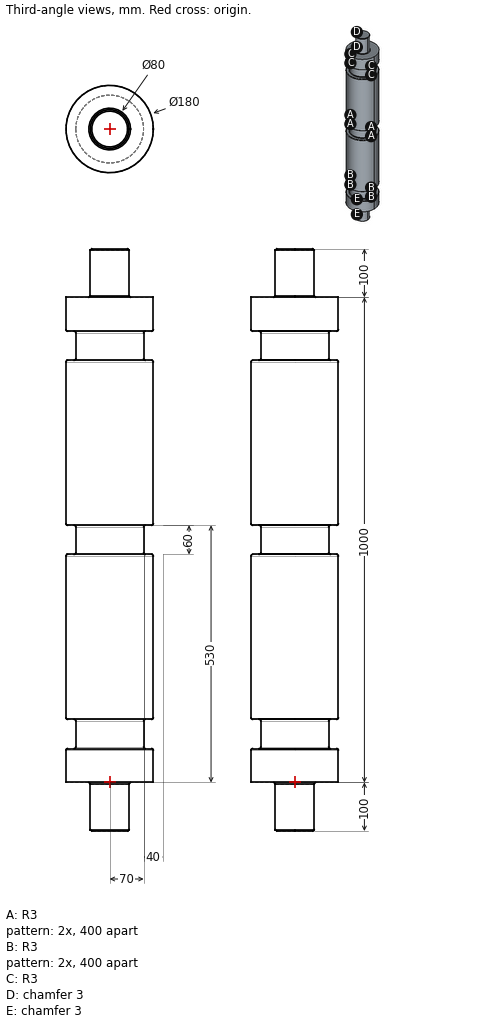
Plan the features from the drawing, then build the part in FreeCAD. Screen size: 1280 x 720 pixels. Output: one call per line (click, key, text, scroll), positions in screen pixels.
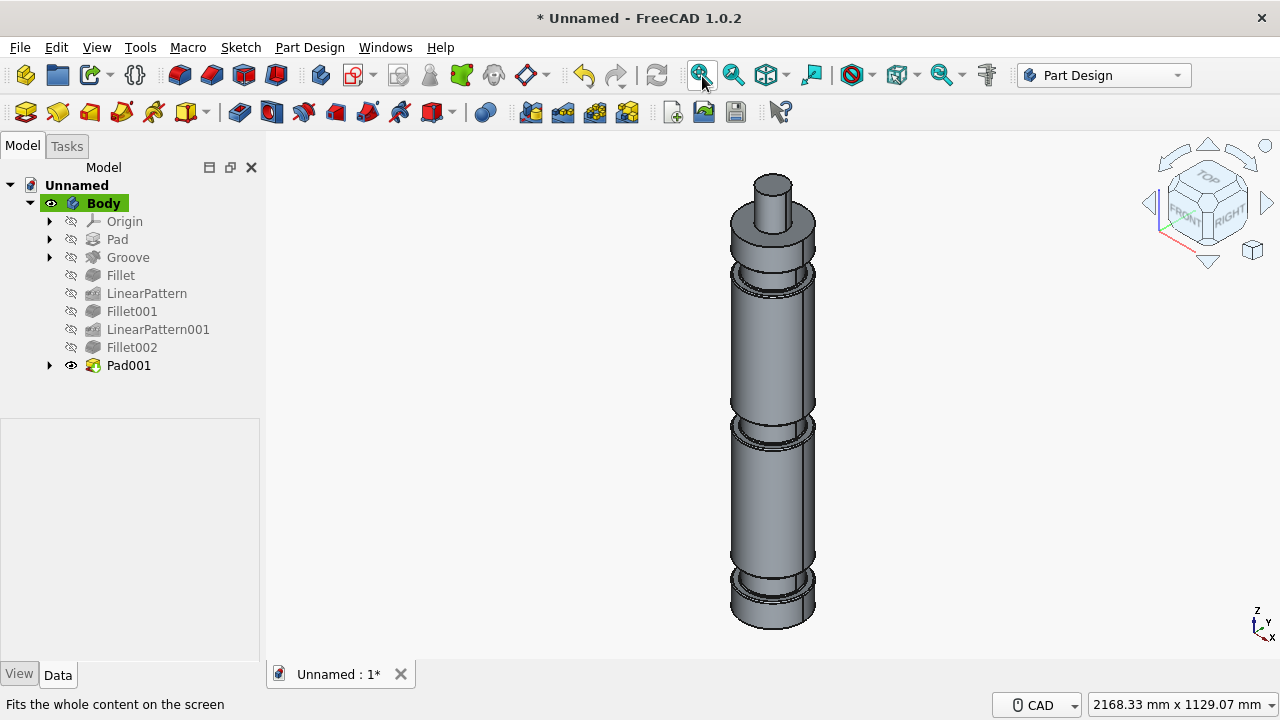
click(756, 227)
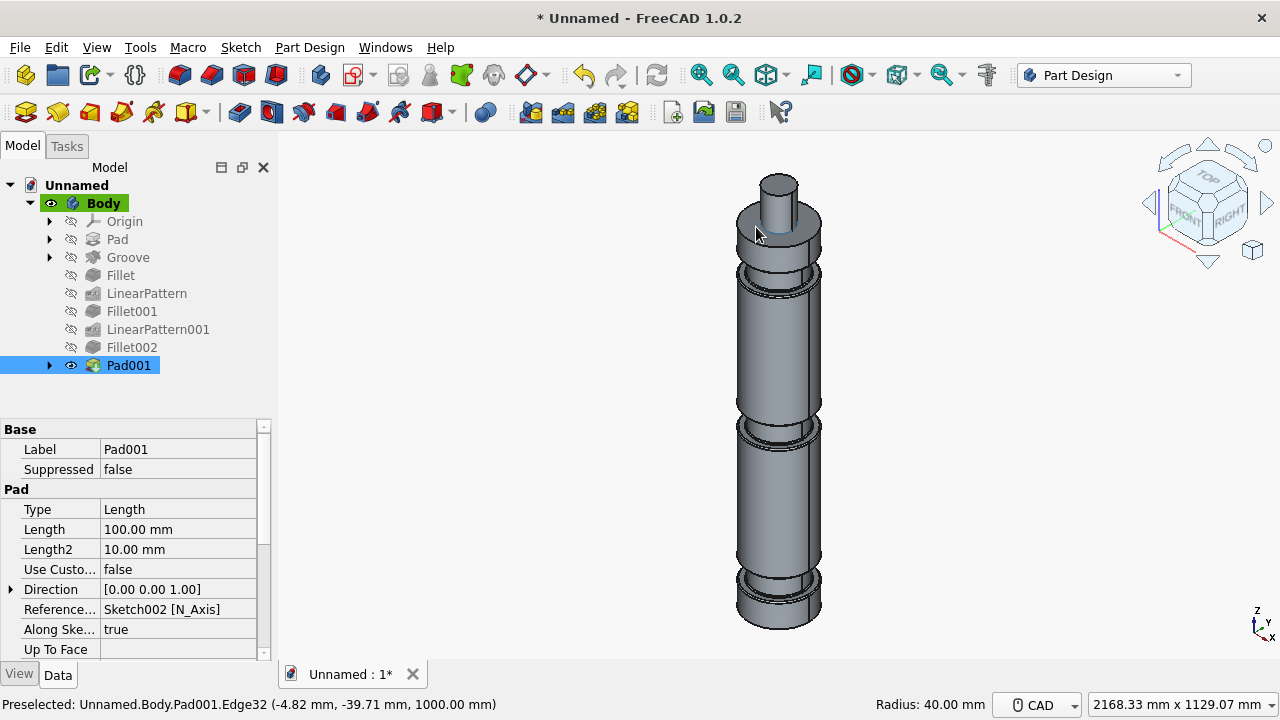
click(761, 182, ctrl)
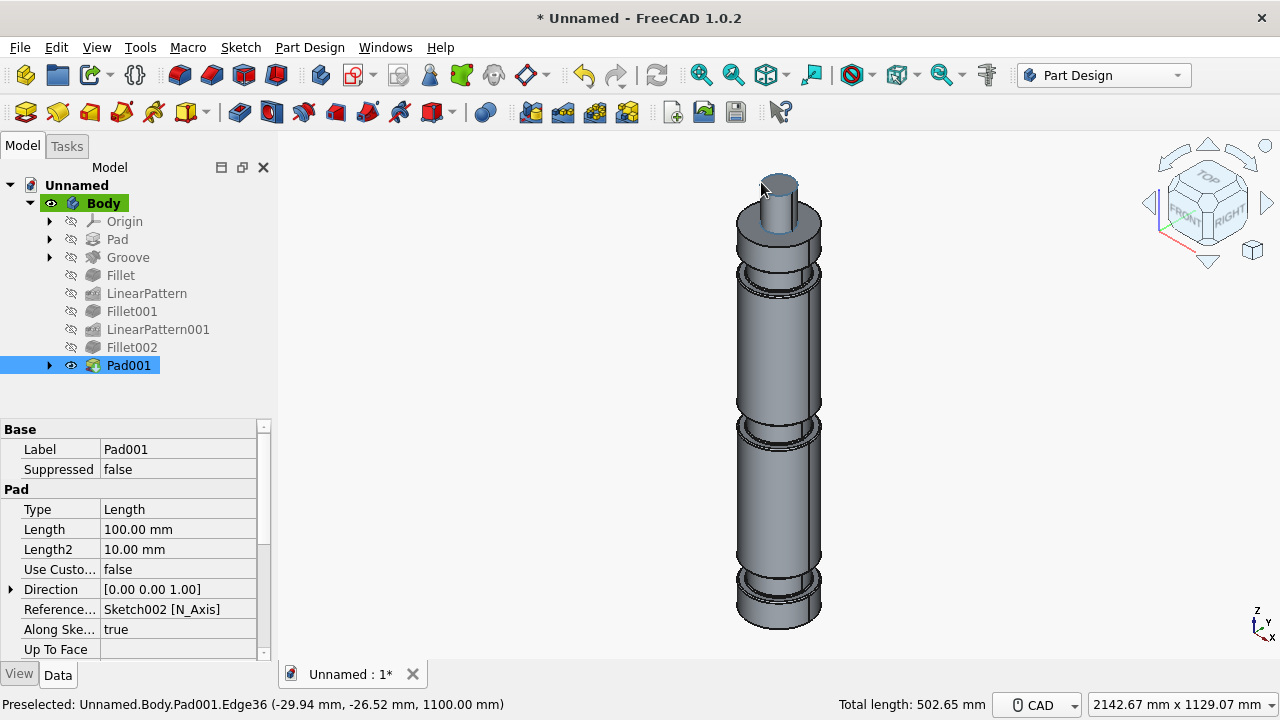
click(212, 76)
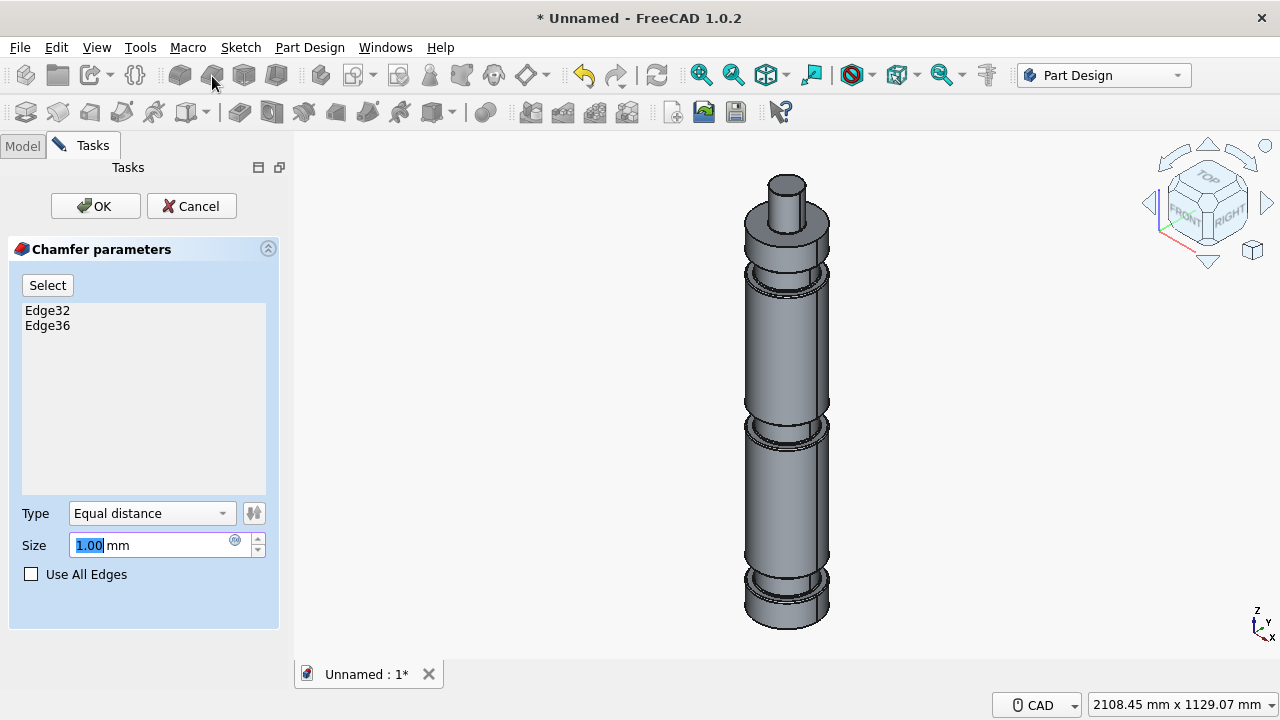
text(3)
key(Tab)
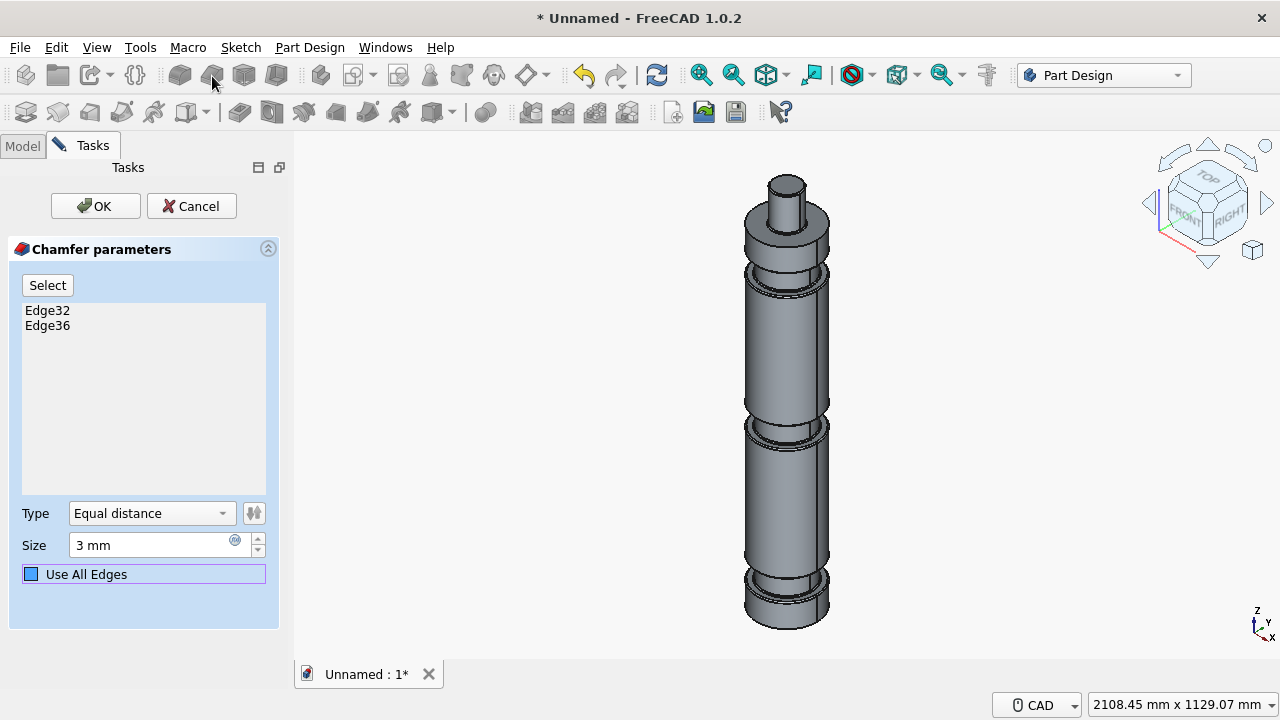
click(96, 206)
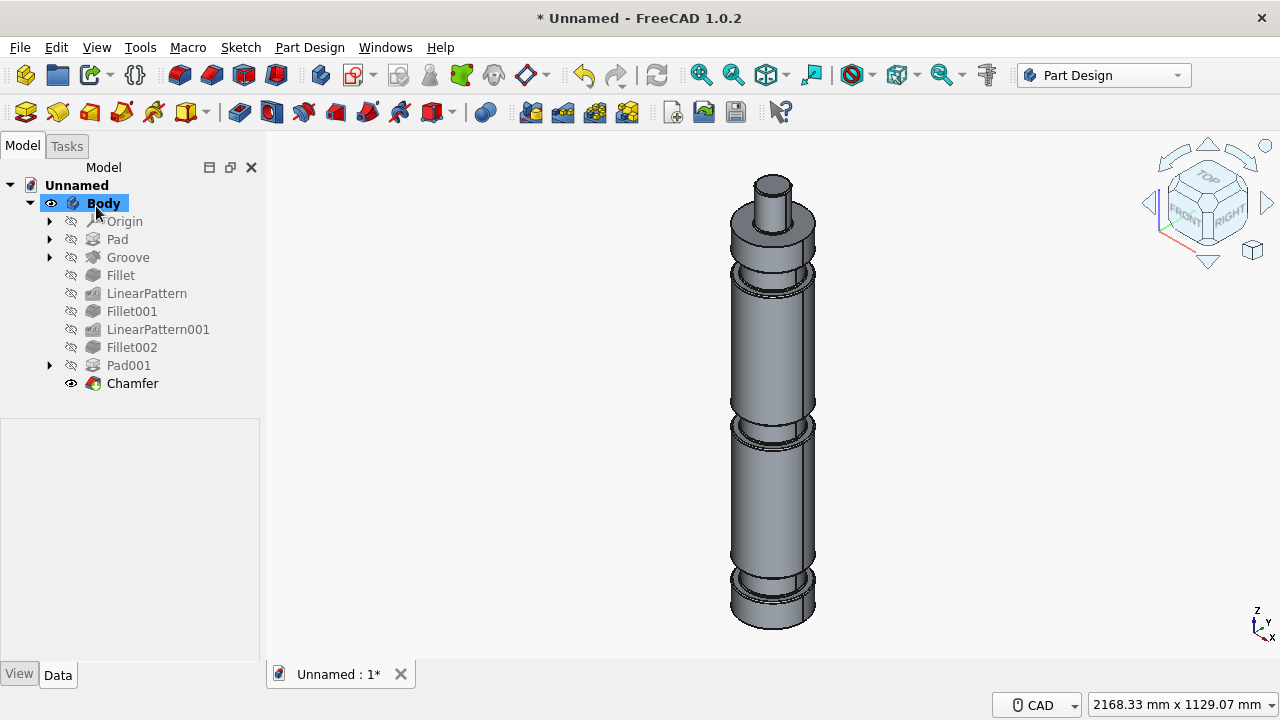
click(50, 221)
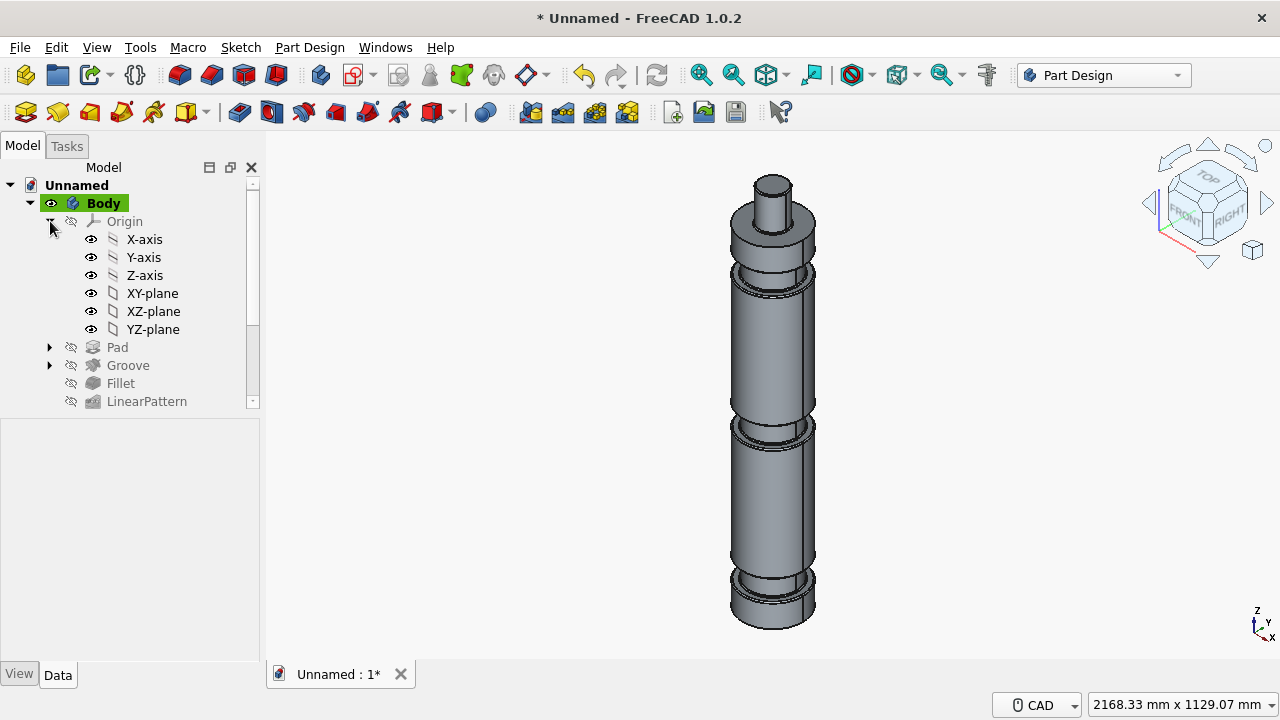
click(136, 293)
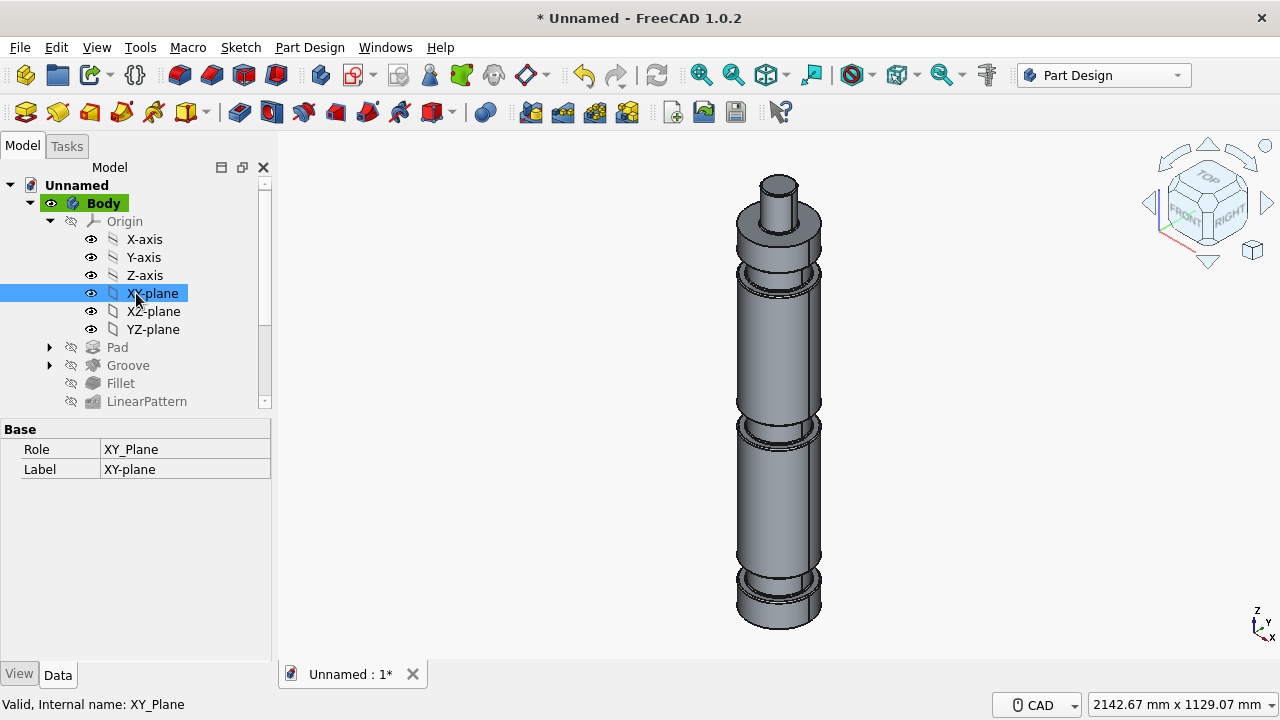
click(526, 76)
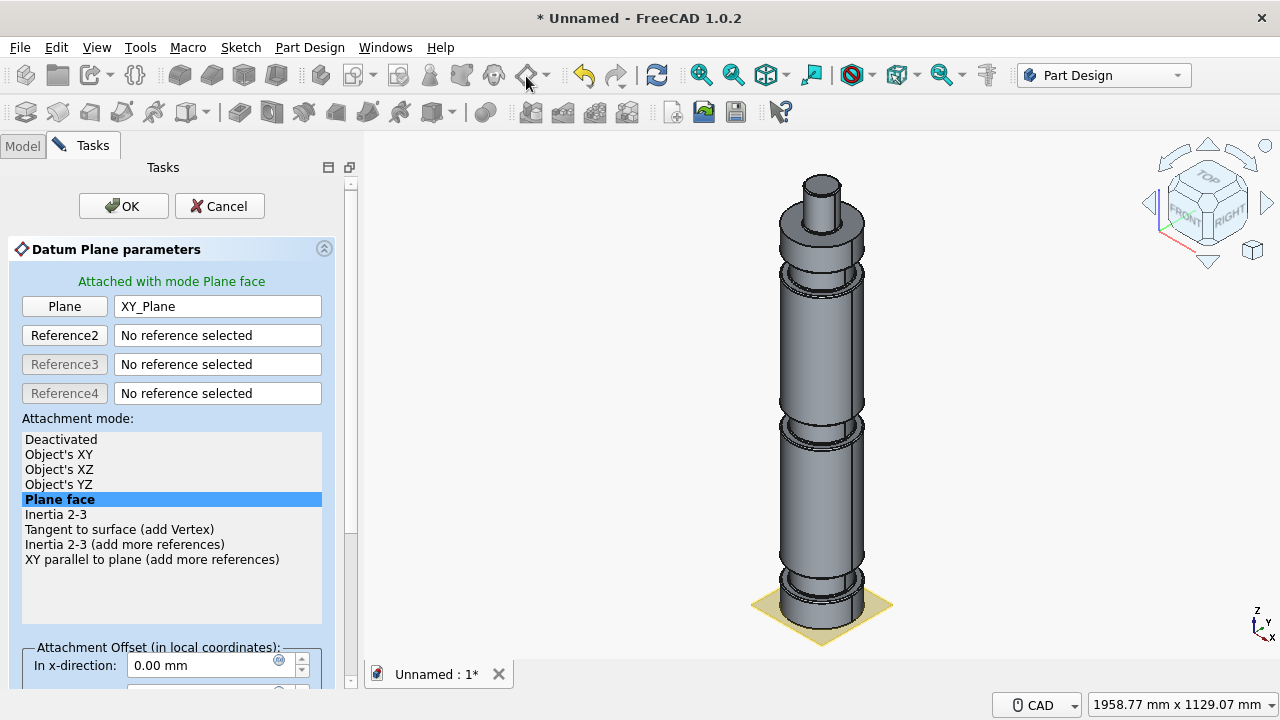
scroll(351, 432, down, 2)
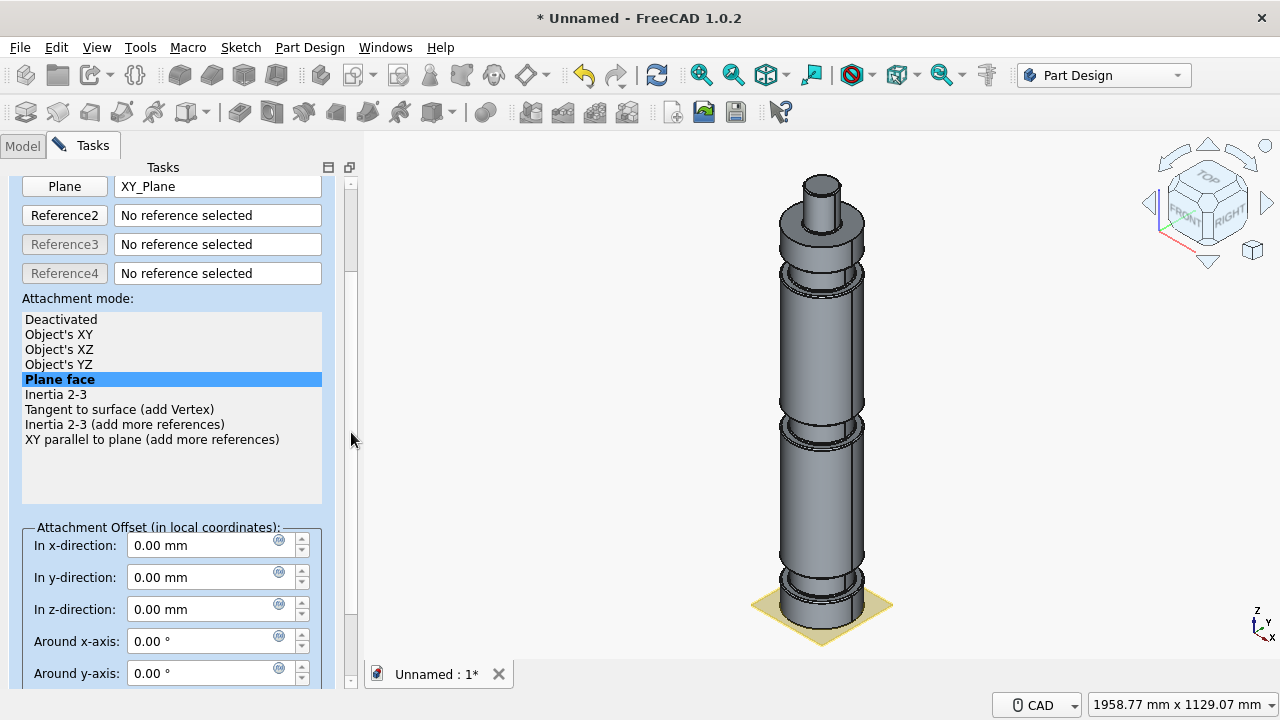
triple_click(210, 609)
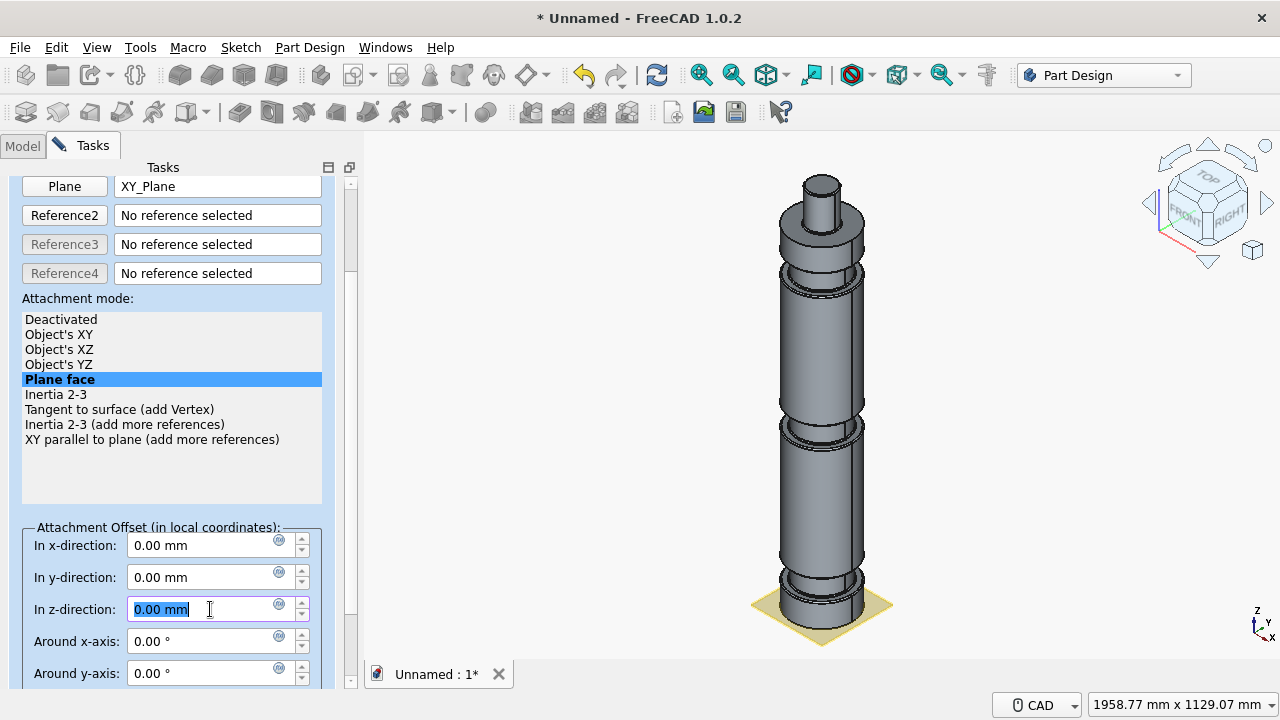
text(-100)
key(Tab)